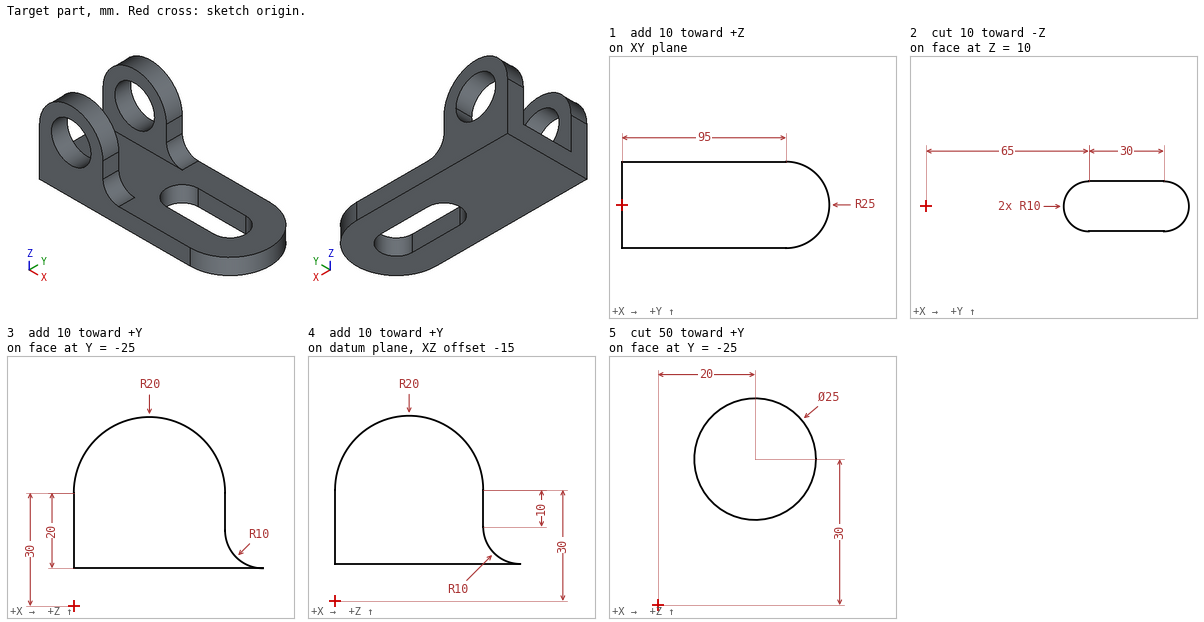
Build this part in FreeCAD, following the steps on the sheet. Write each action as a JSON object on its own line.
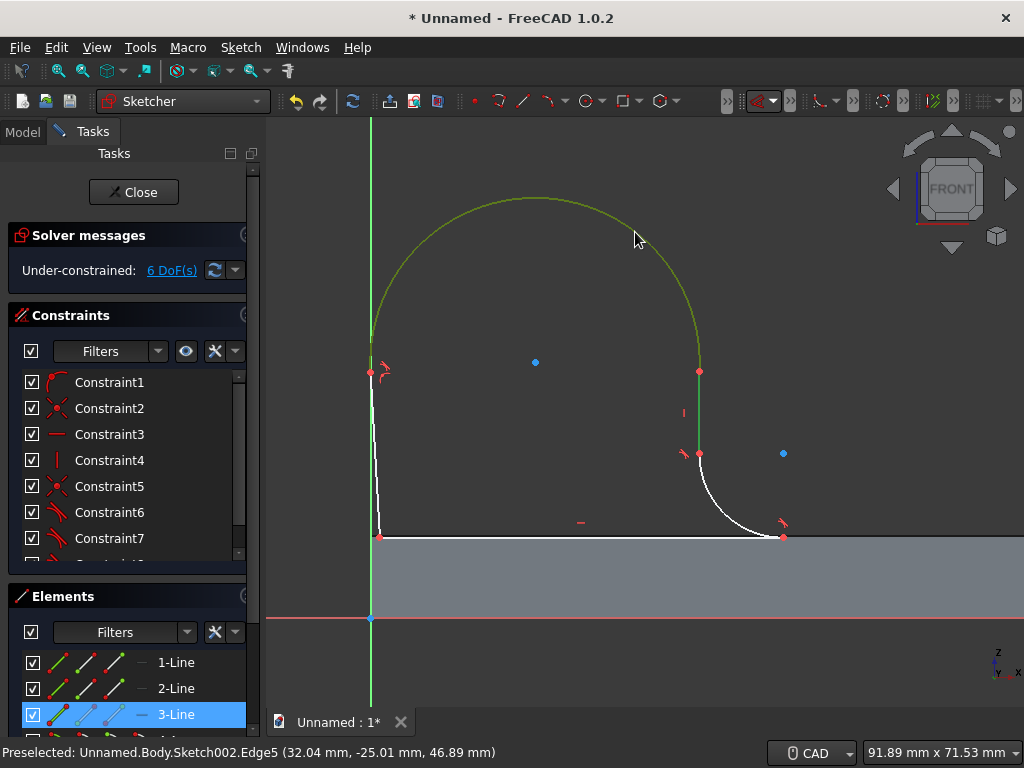
{"action": "key", "text": "t"}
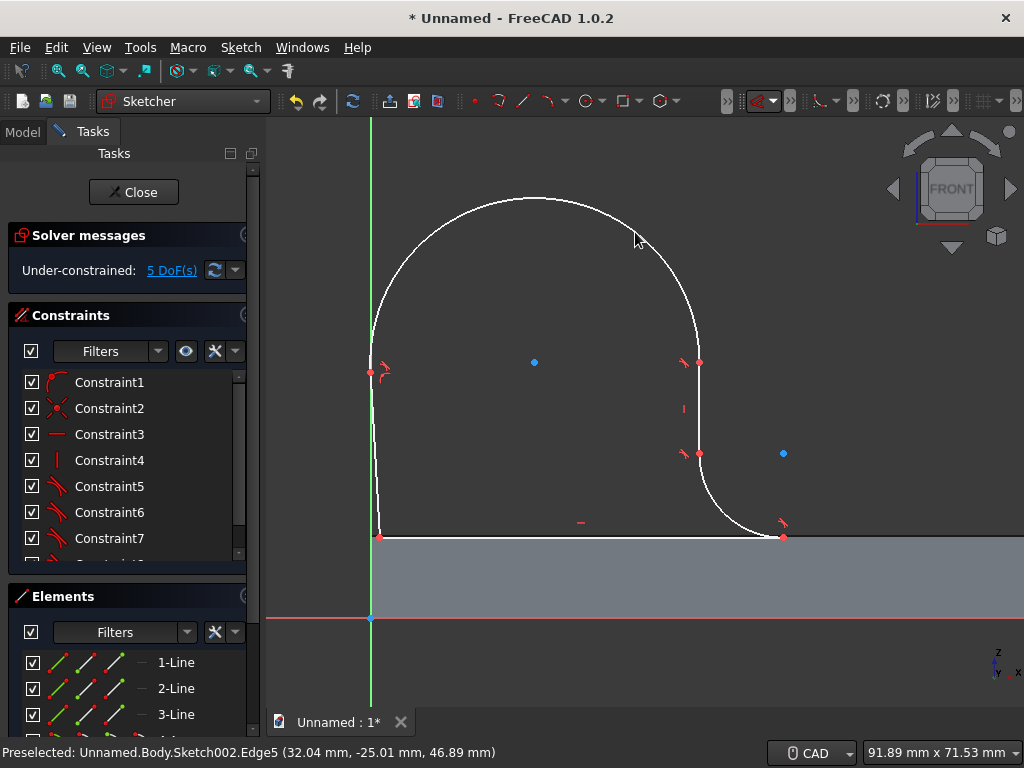
{"action": "left_click", "coordinate": [373, 422]}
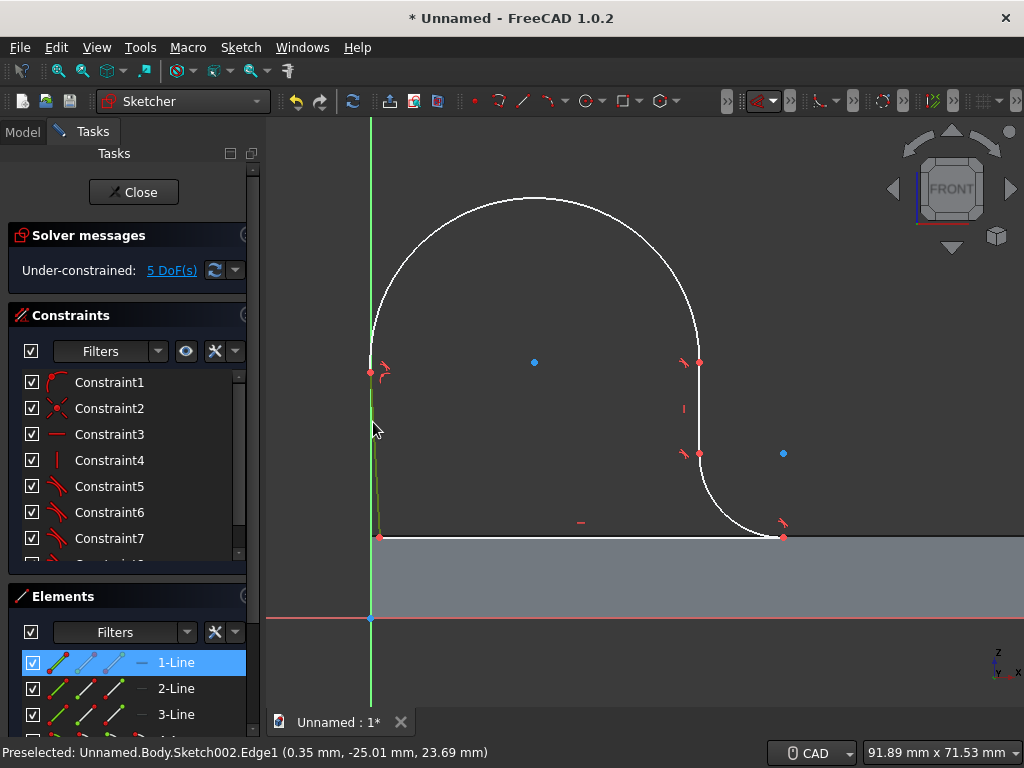
{"action": "key", "text": "v"}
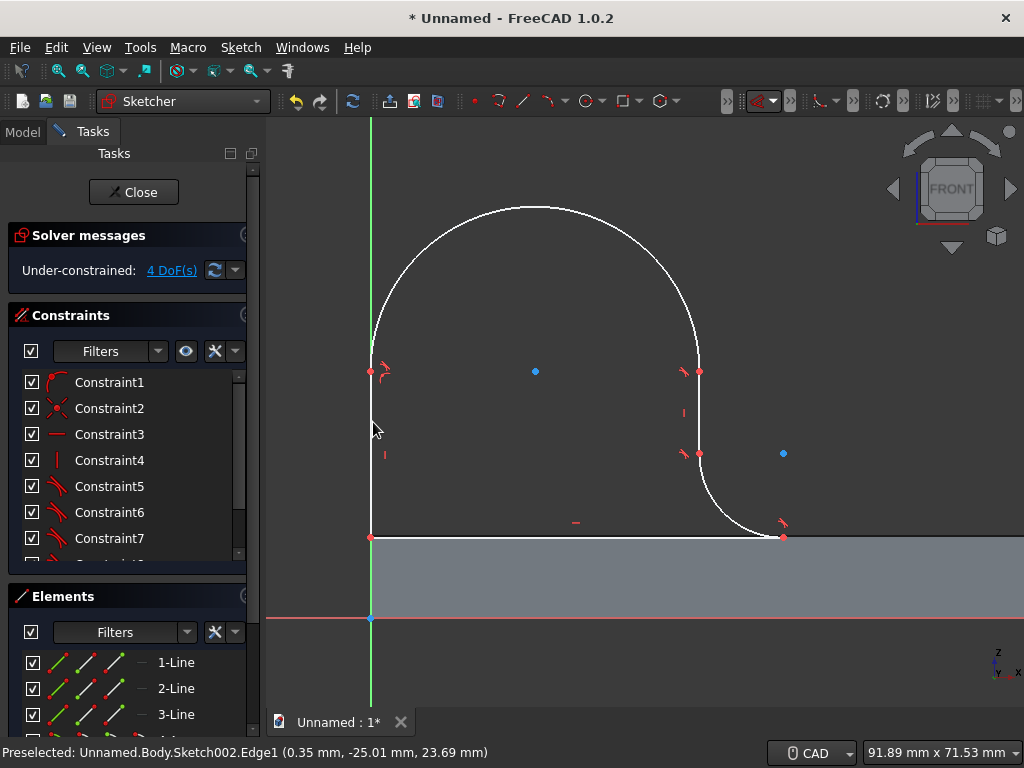
{"action": "left_click", "coordinate": [709, 492]}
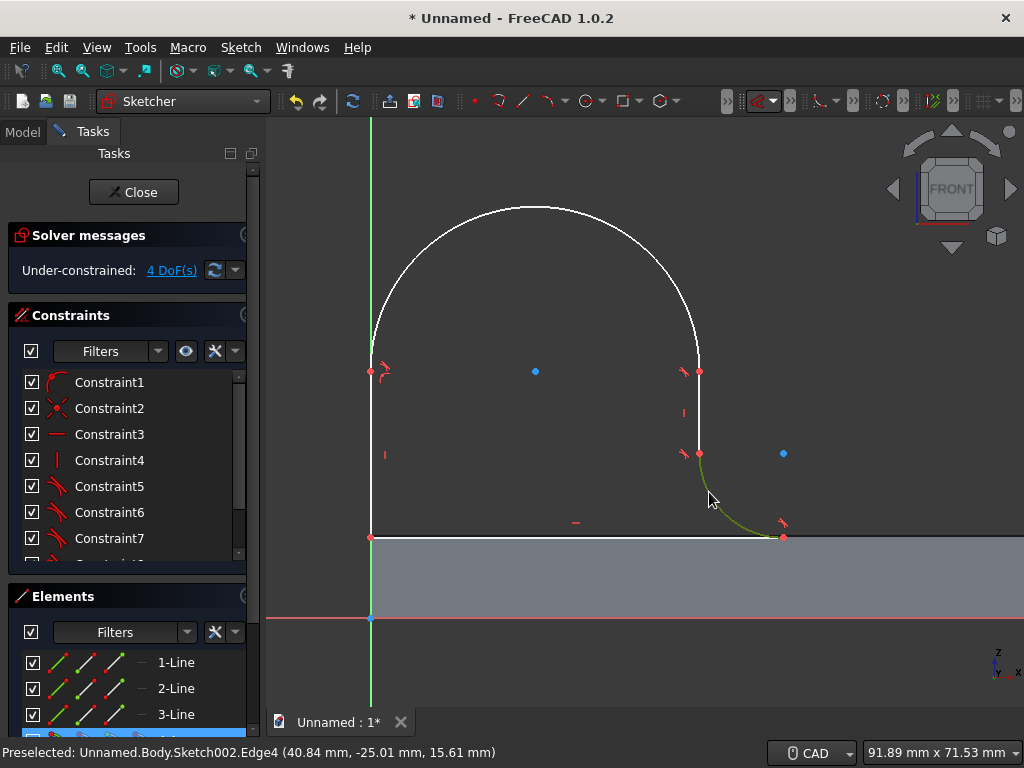
{"action": "left_click", "coordinate": [776, 102]}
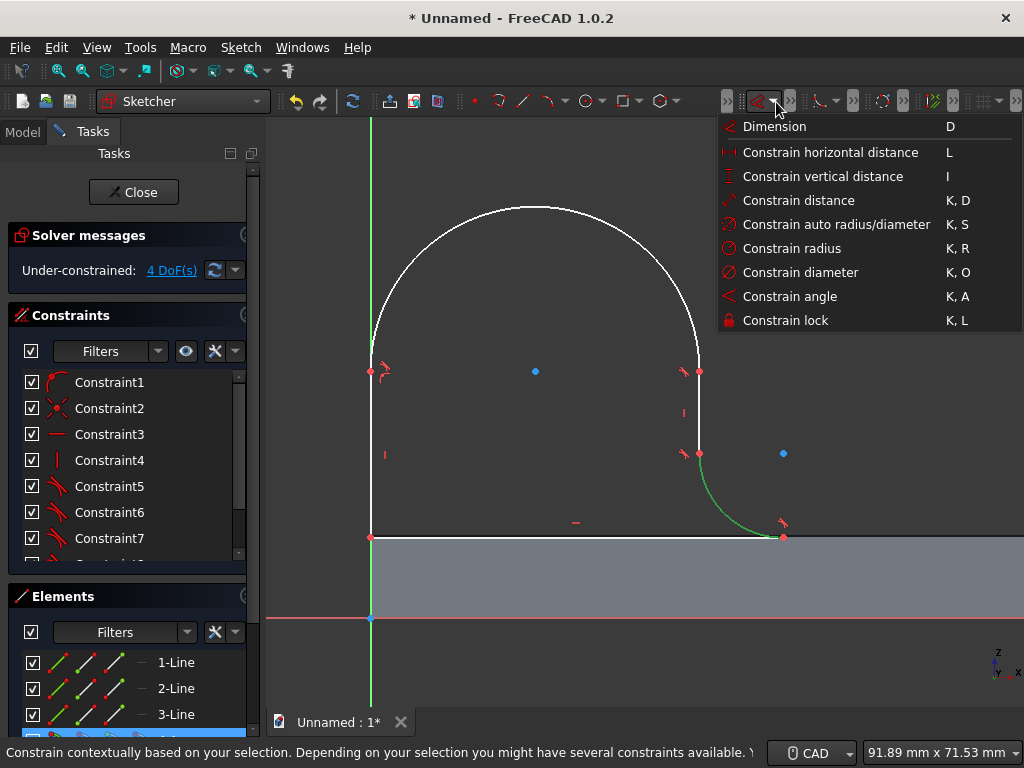
{"action": "left_click", "coordinate": [870, 248]}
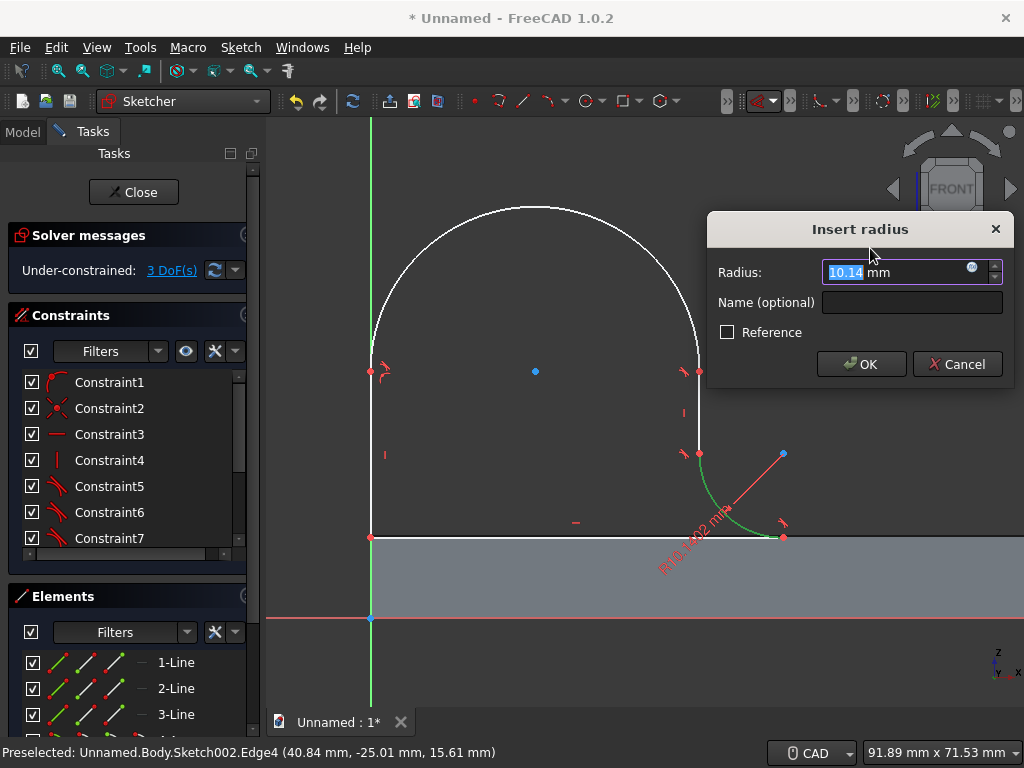
{"action": "type", "text": "10"}
{"action": "key", "text": "Return"}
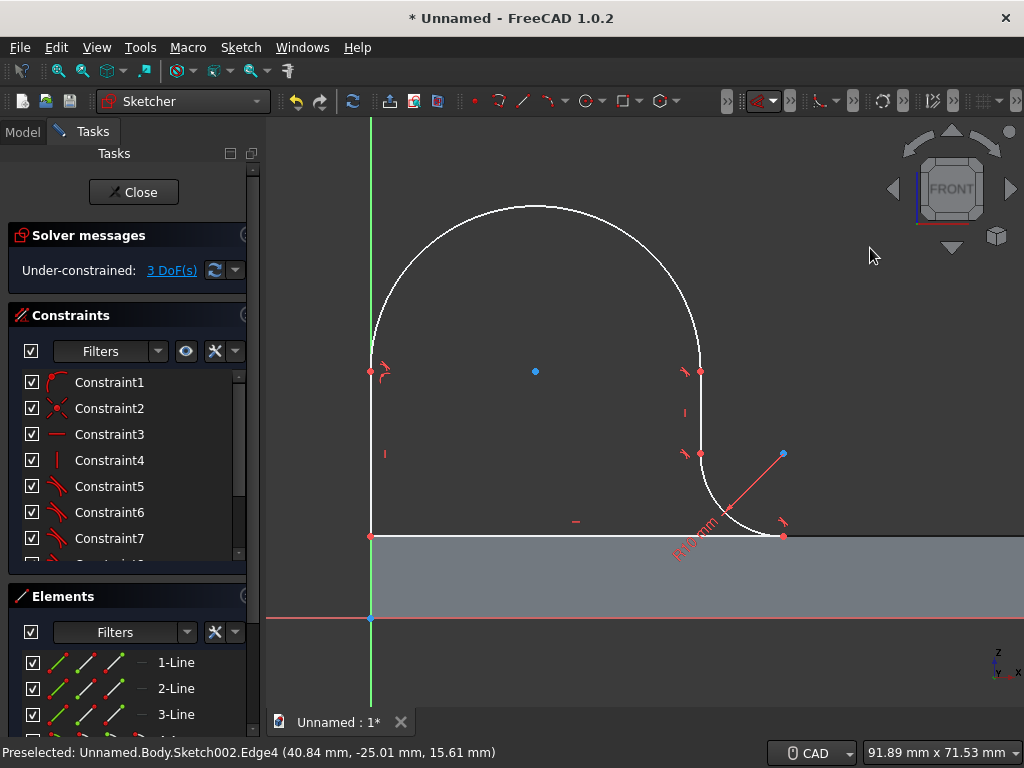
{"action": "left_click", "coordinate": [633, 238]}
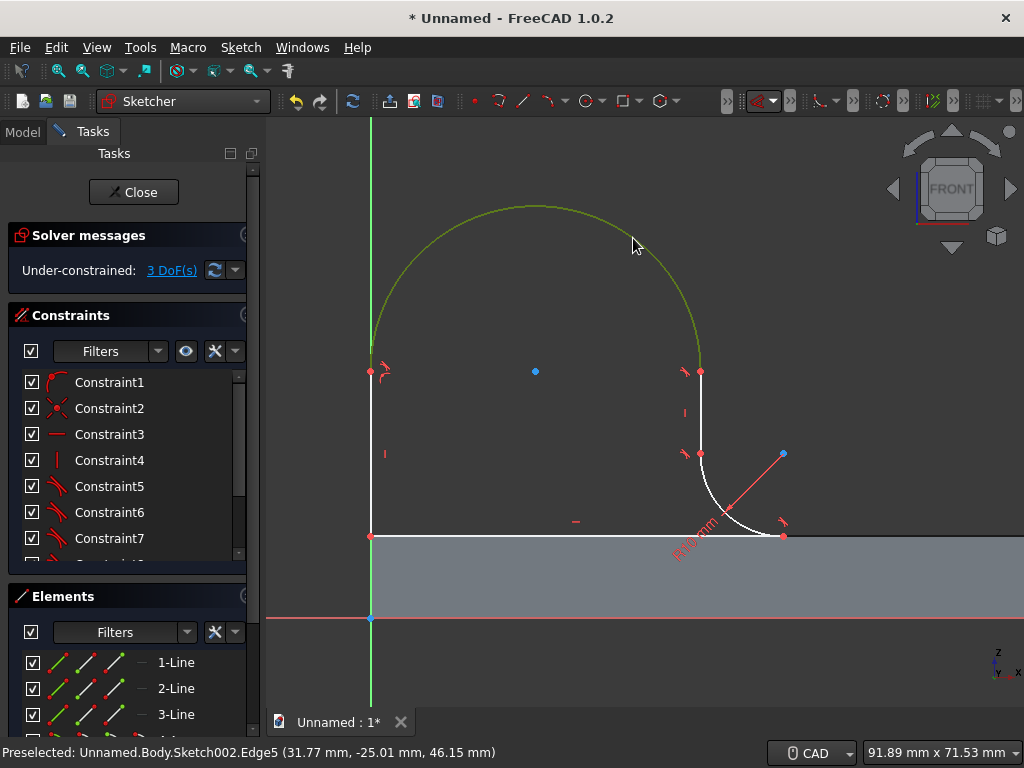
{"action": "left_click", "coordinate": [776, 102]}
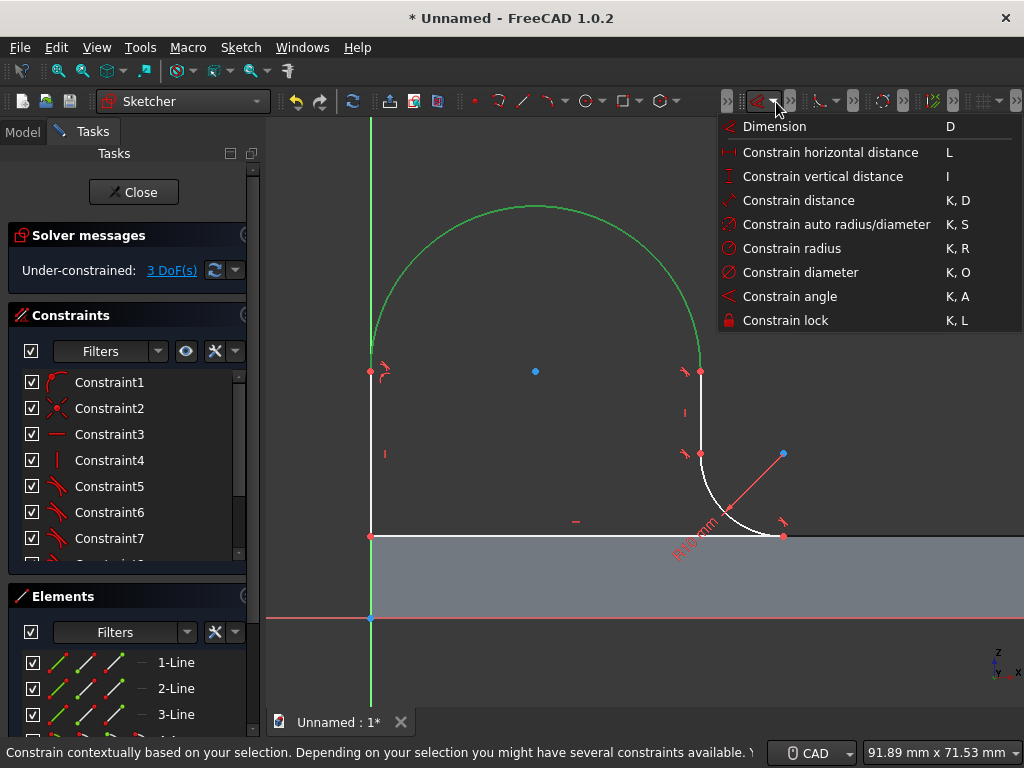
{"action": "left_click", "coordinate": [870, 248]}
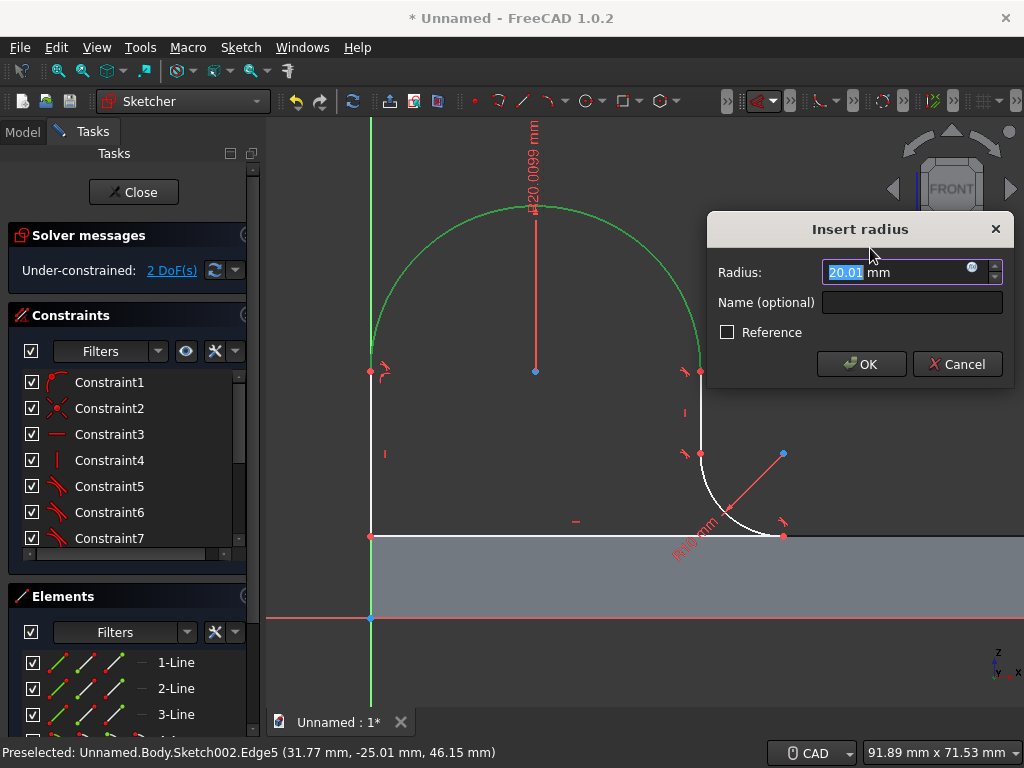
{"action": "type", "text": "20"}
{"action": "key", "text": "Return"}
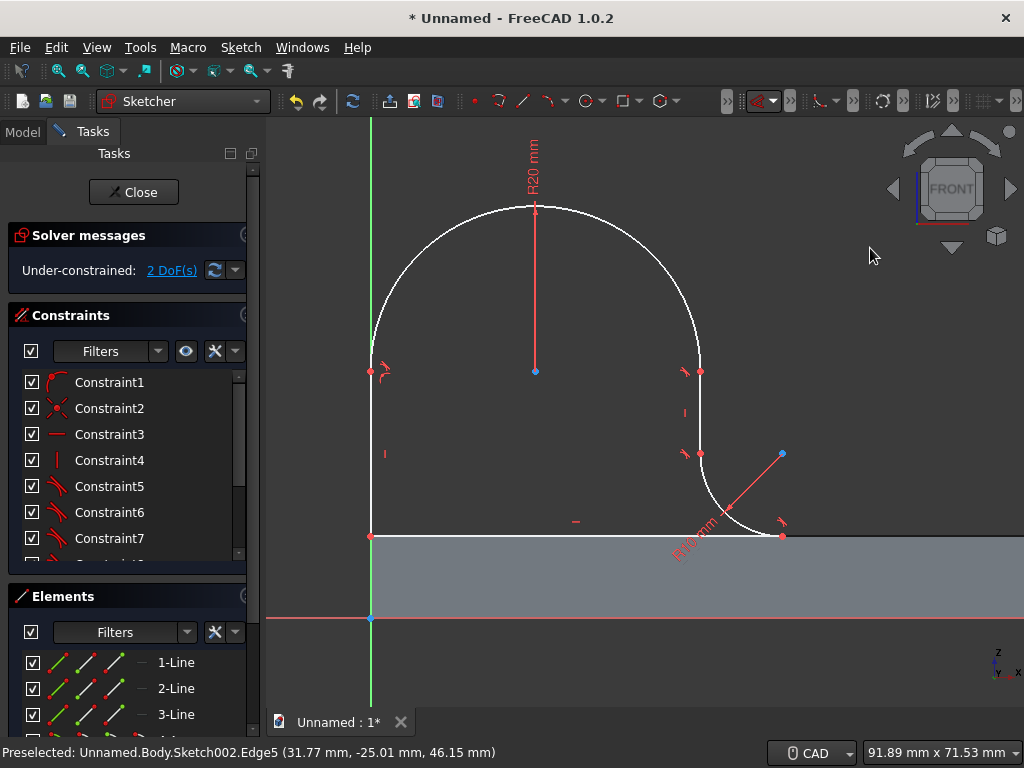
{"action": "left_click", "coordinate": [371, 421]}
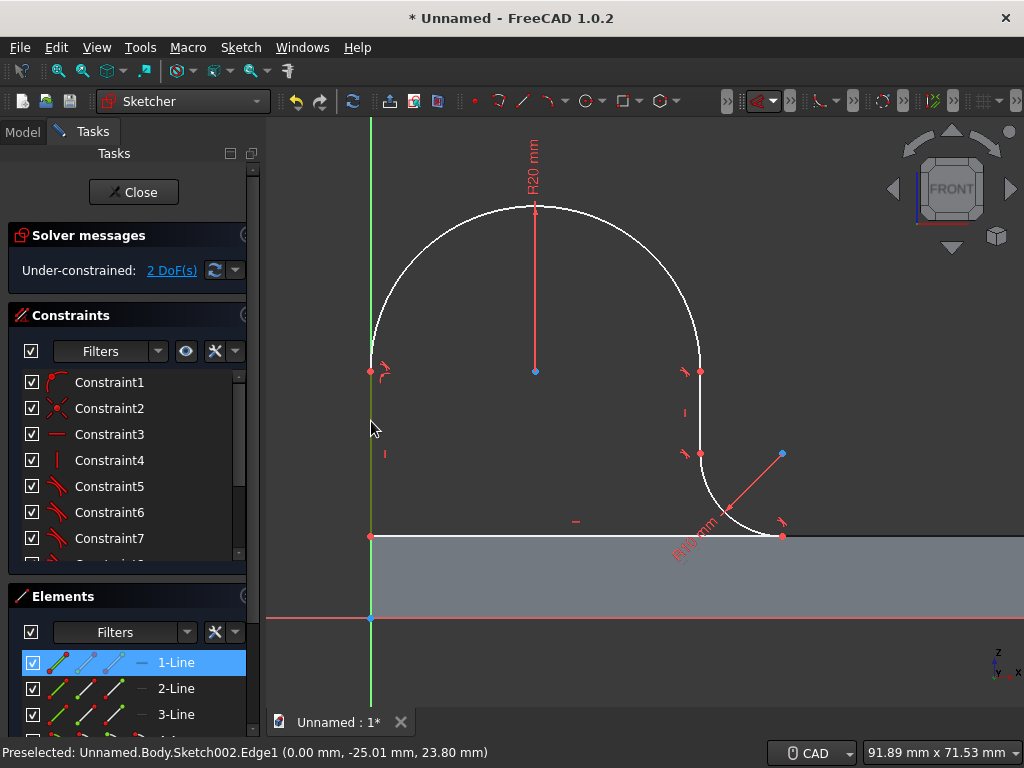
{"action": "left_click", "coordinate": [776, 102]}